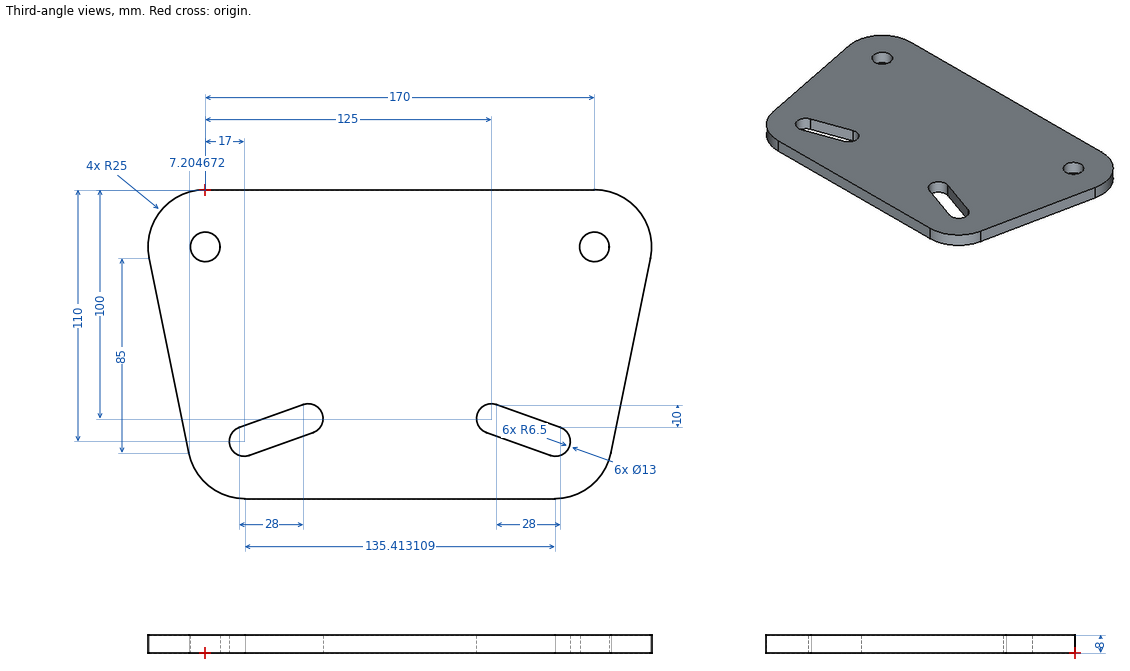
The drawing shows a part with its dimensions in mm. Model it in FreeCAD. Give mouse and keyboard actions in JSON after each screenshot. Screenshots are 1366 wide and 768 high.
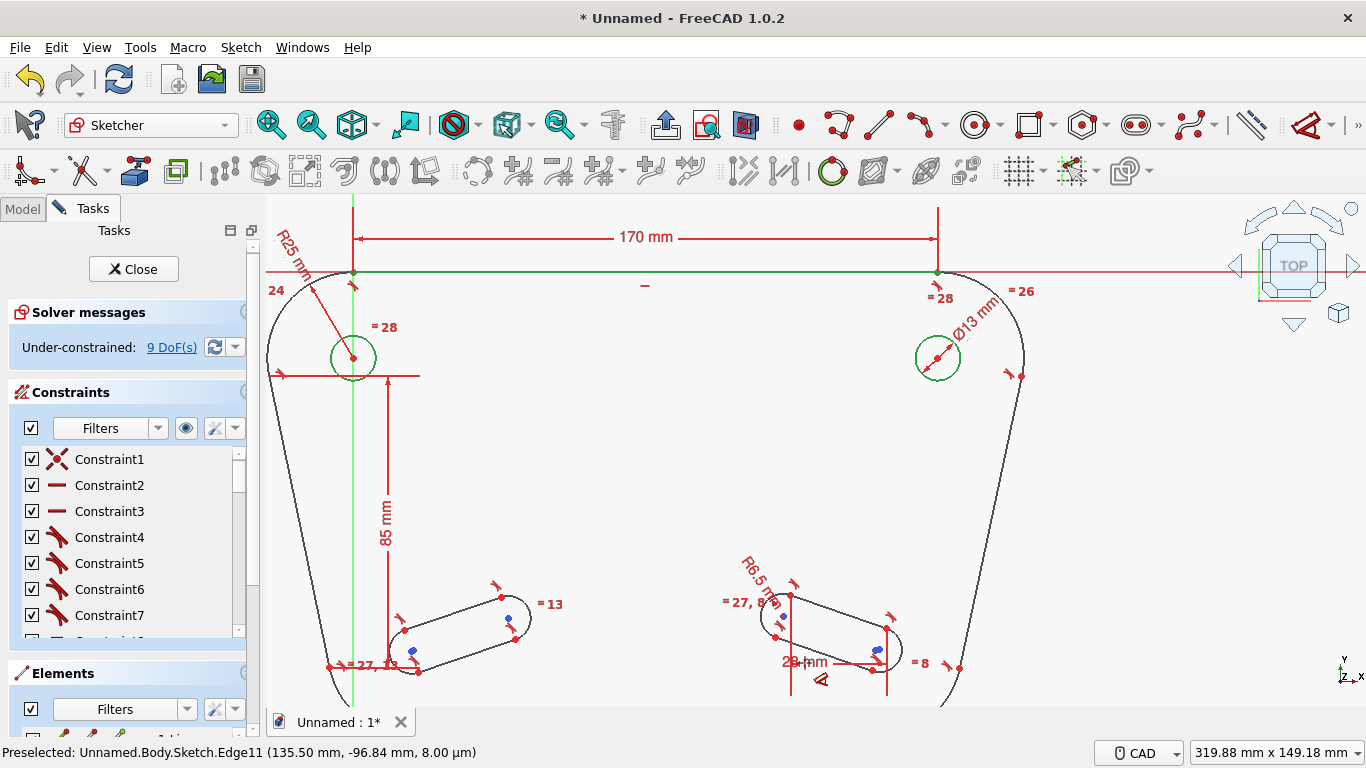
{"action": "left_click", "coordinate": [819, 605]}
{"action": "left_click", "coordinate": [921, 612]}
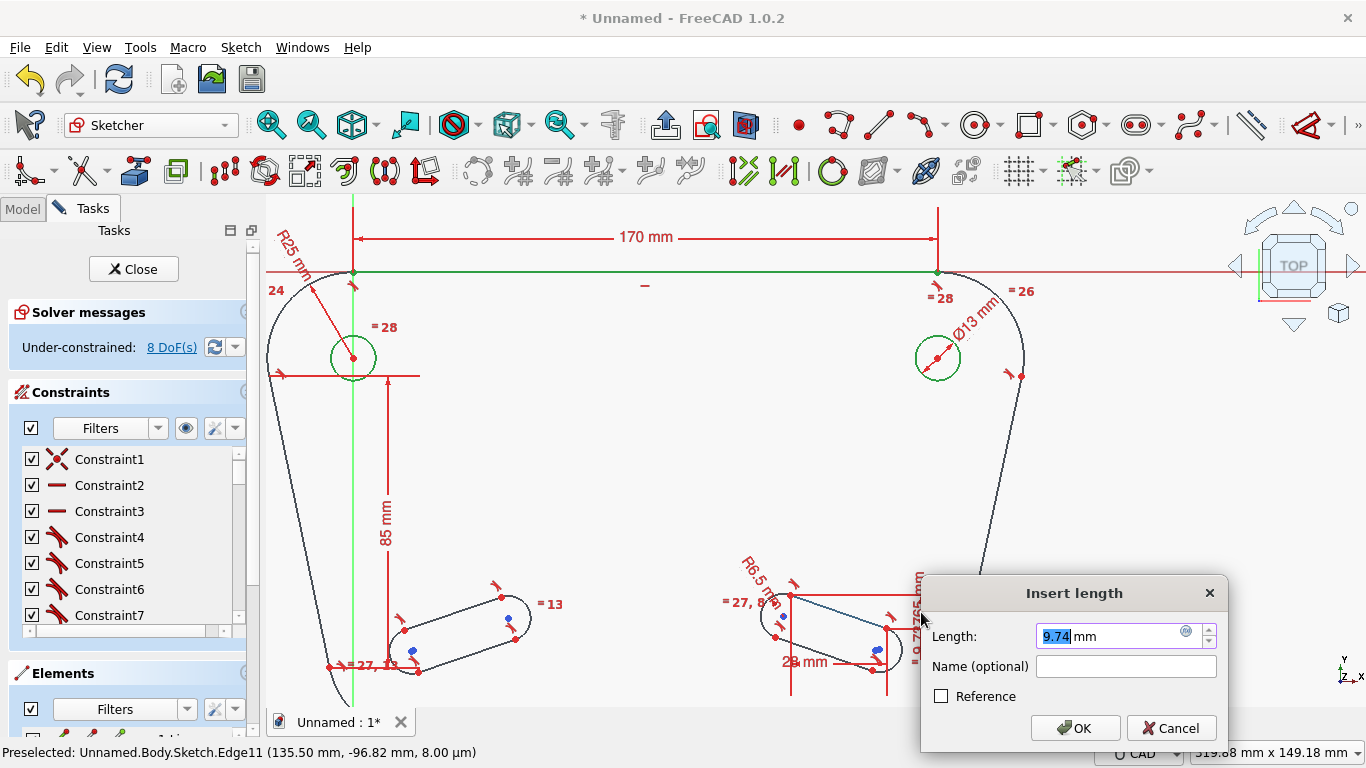
{"action": "type", "text": "10"}
{"action": "key", "text": "Return"}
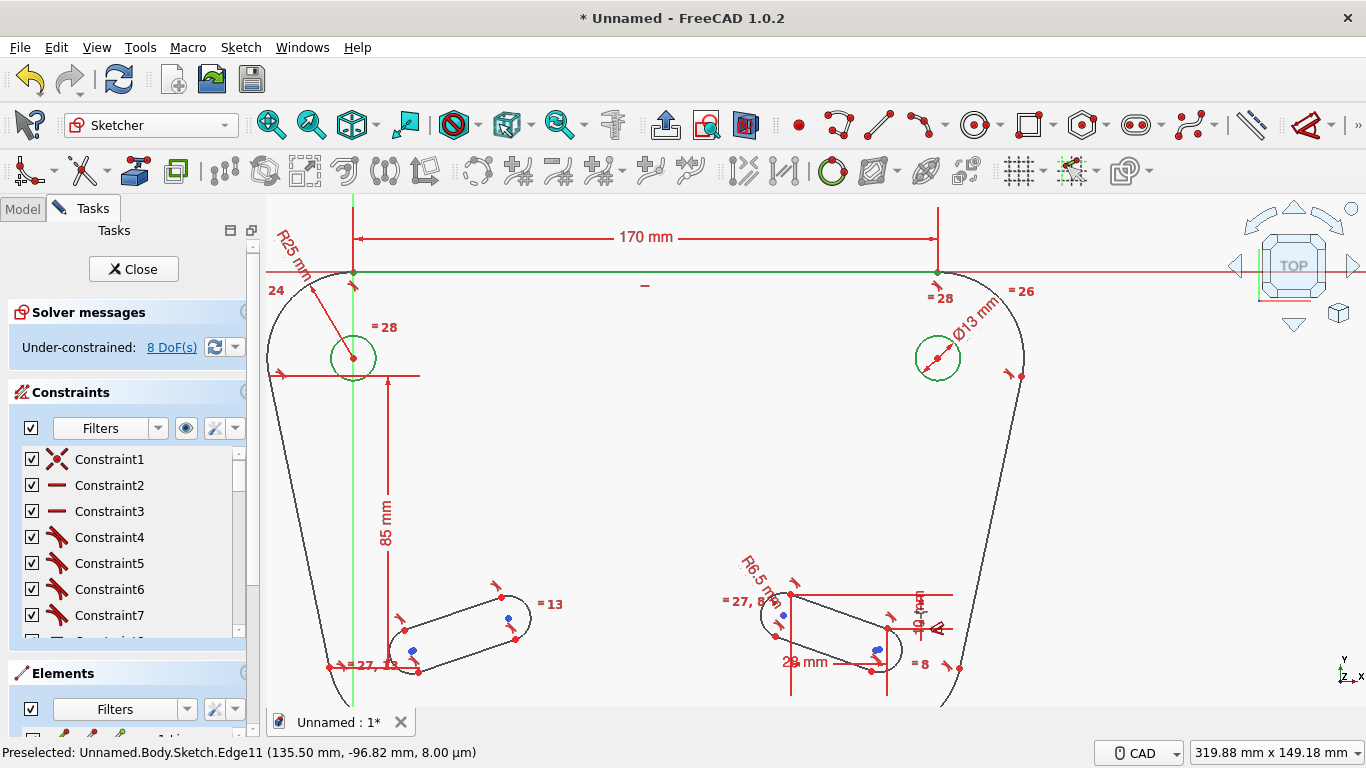
{"action": "left_click", "coordinate": [433, 620]}
{"action": "left_click", "coordinate": [487, 664]}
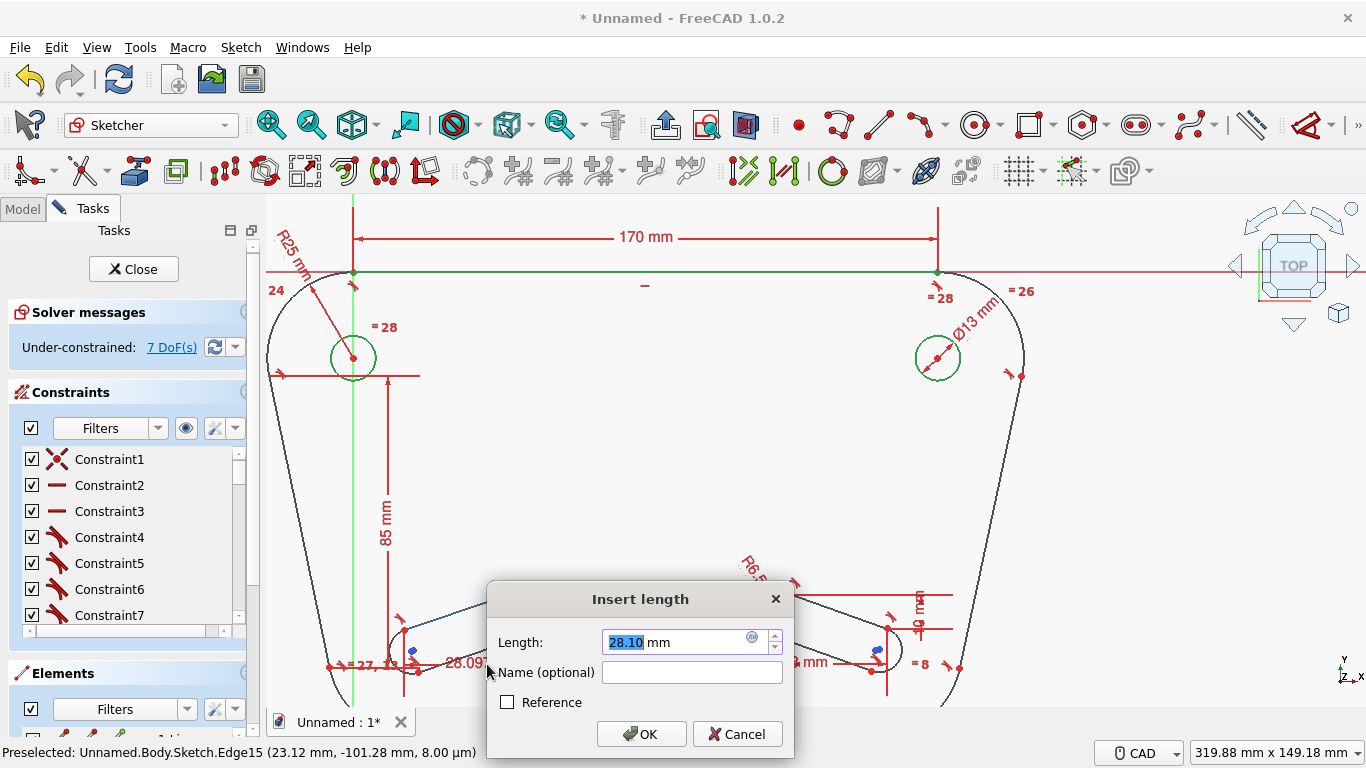
{"action": "type", "text": "28"}
{"action": "key", "text": "Return"}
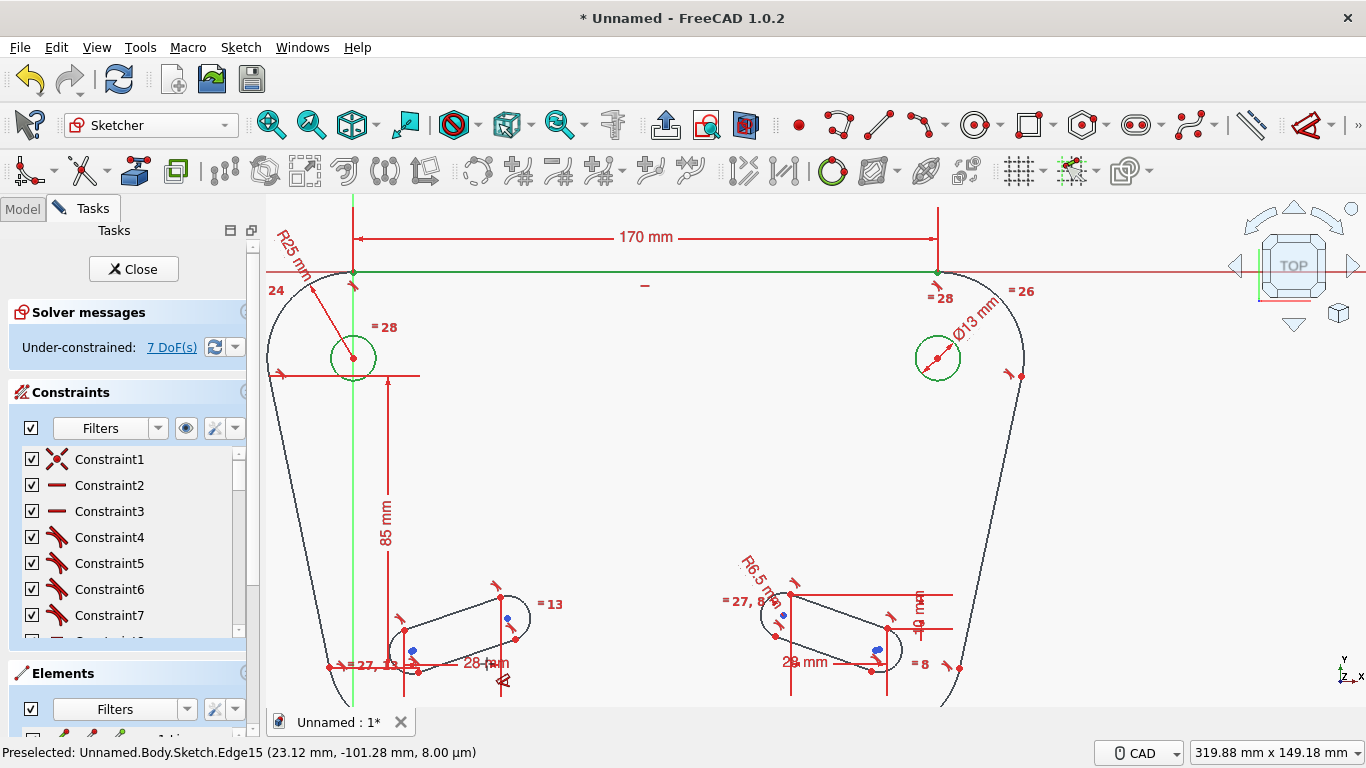
{"action": "left_click", "coordinate": [433, 620]}
{"action": "left_click", "coordinate": [370, 614]}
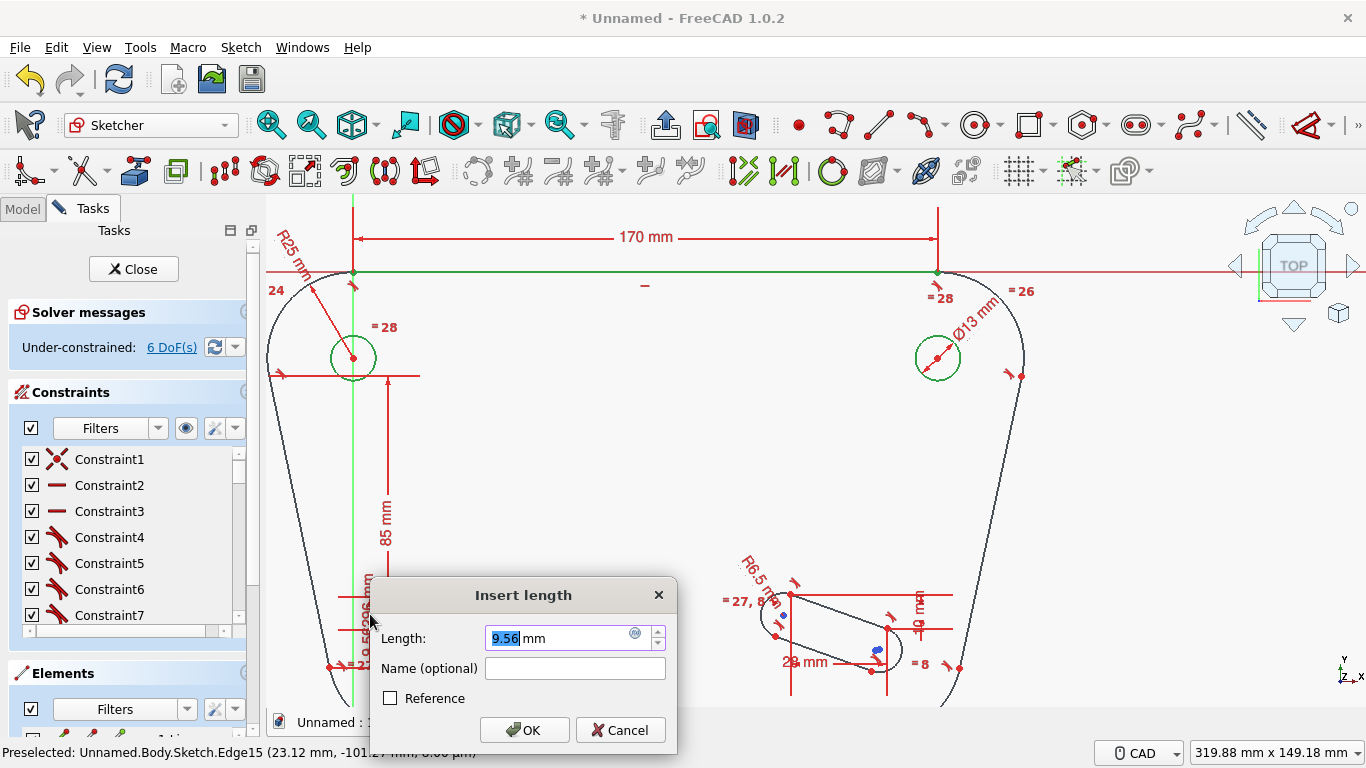
{"action": "type", "text": "10"}
{"action": "key", "text": "Return"}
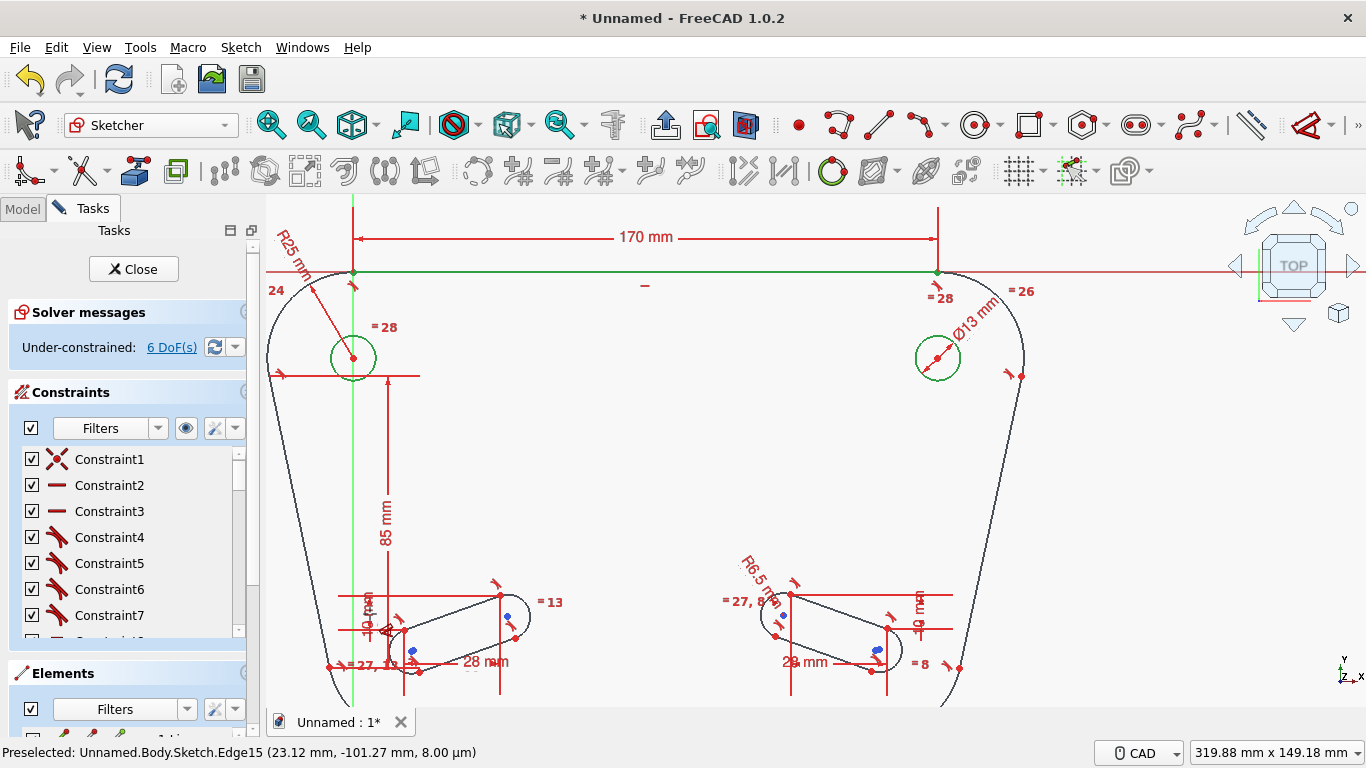
{"action": "scroll", "coordinate": [412, 651], "scroll_direction": "up", "scroll_amount": 9}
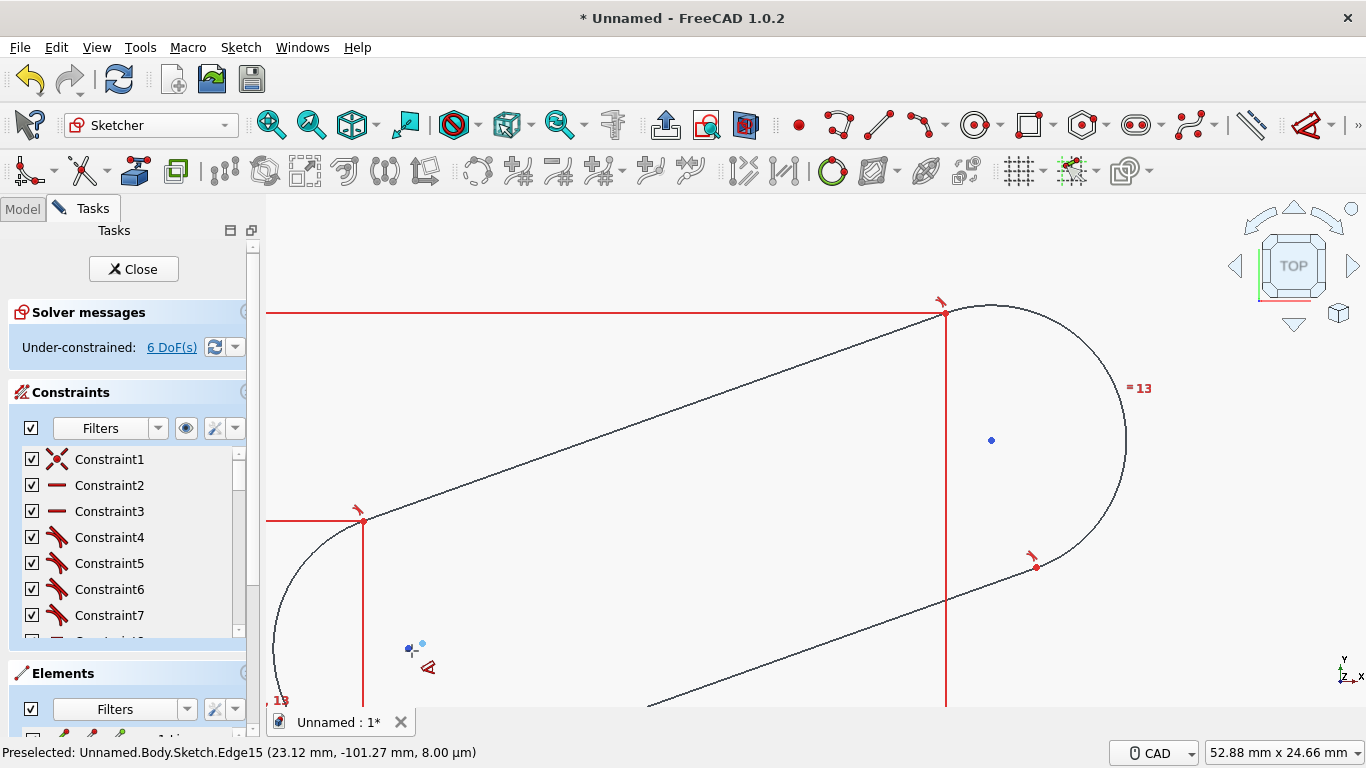
{"action": "left_click", "coordinate": [409, 649]}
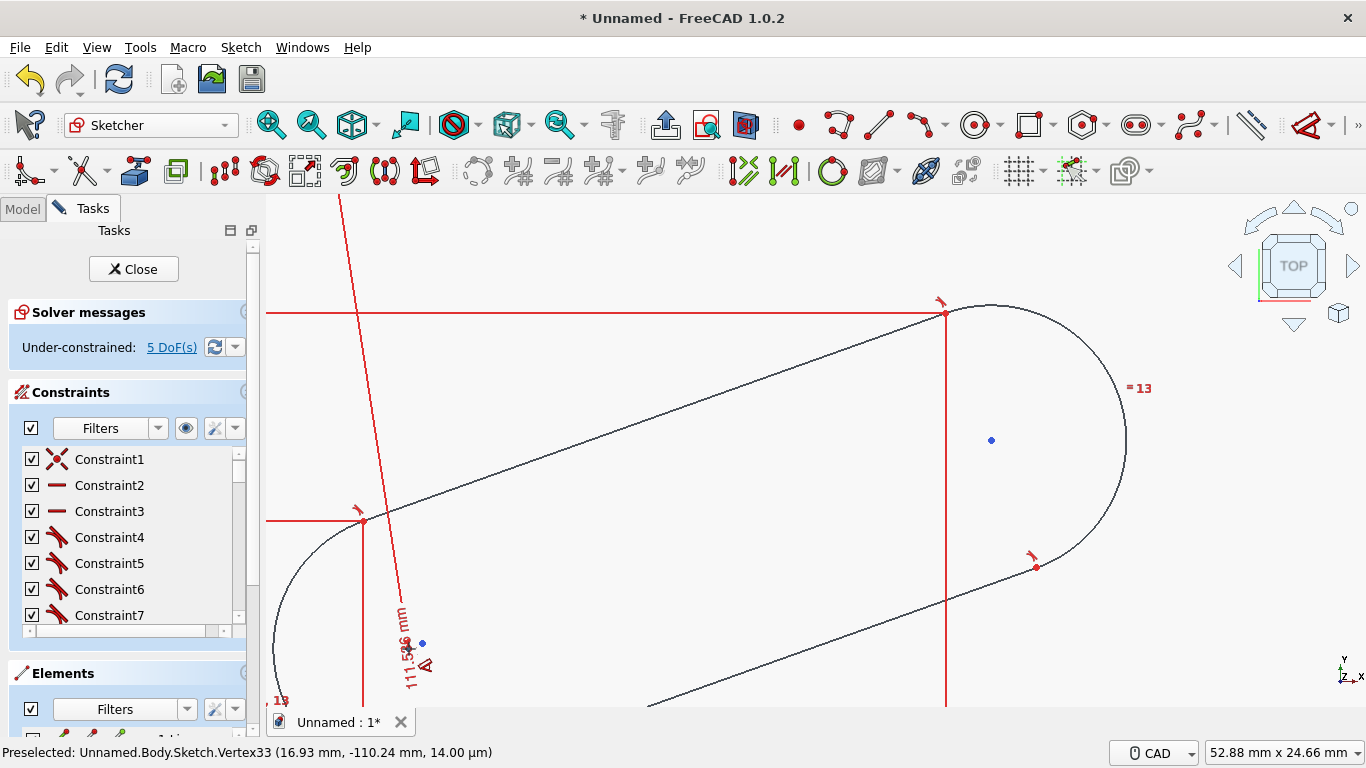
{"action": "key", "text": "Escape"}
{"action": "key", "text": "Escape"}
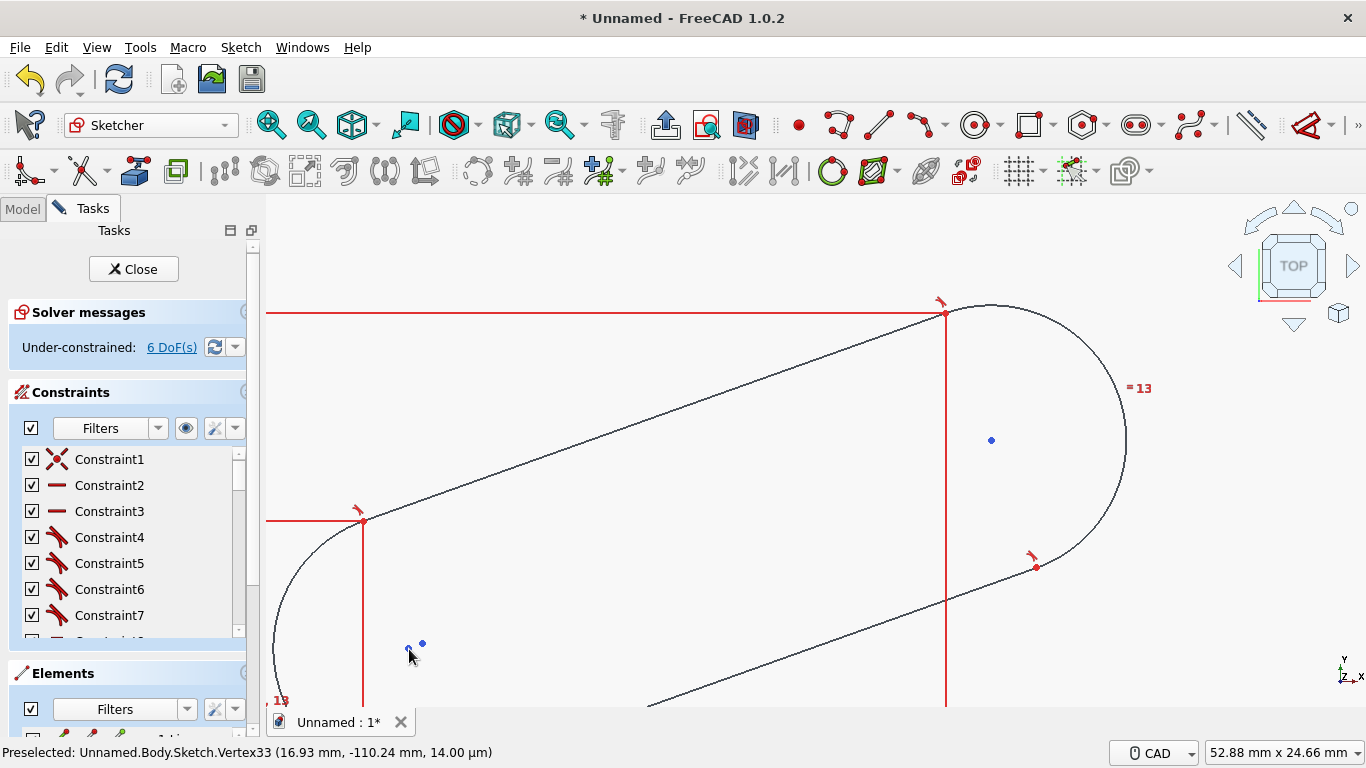
{"action": "left_click", "coordinate": [409, 649]}